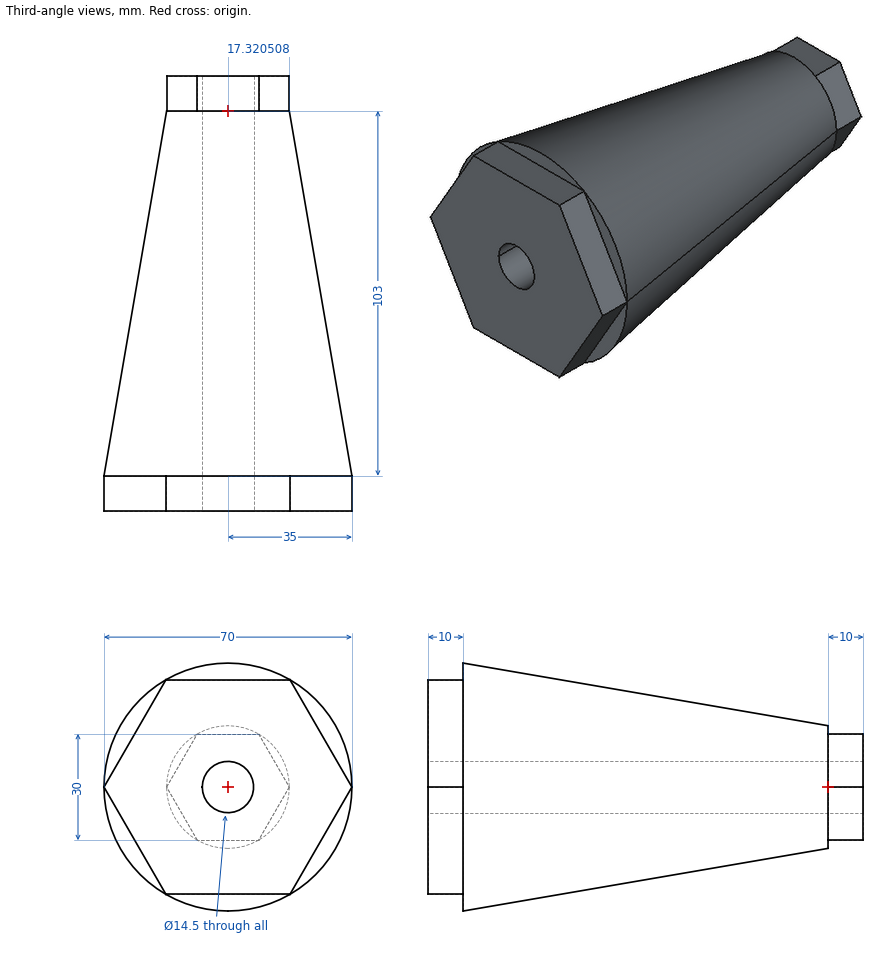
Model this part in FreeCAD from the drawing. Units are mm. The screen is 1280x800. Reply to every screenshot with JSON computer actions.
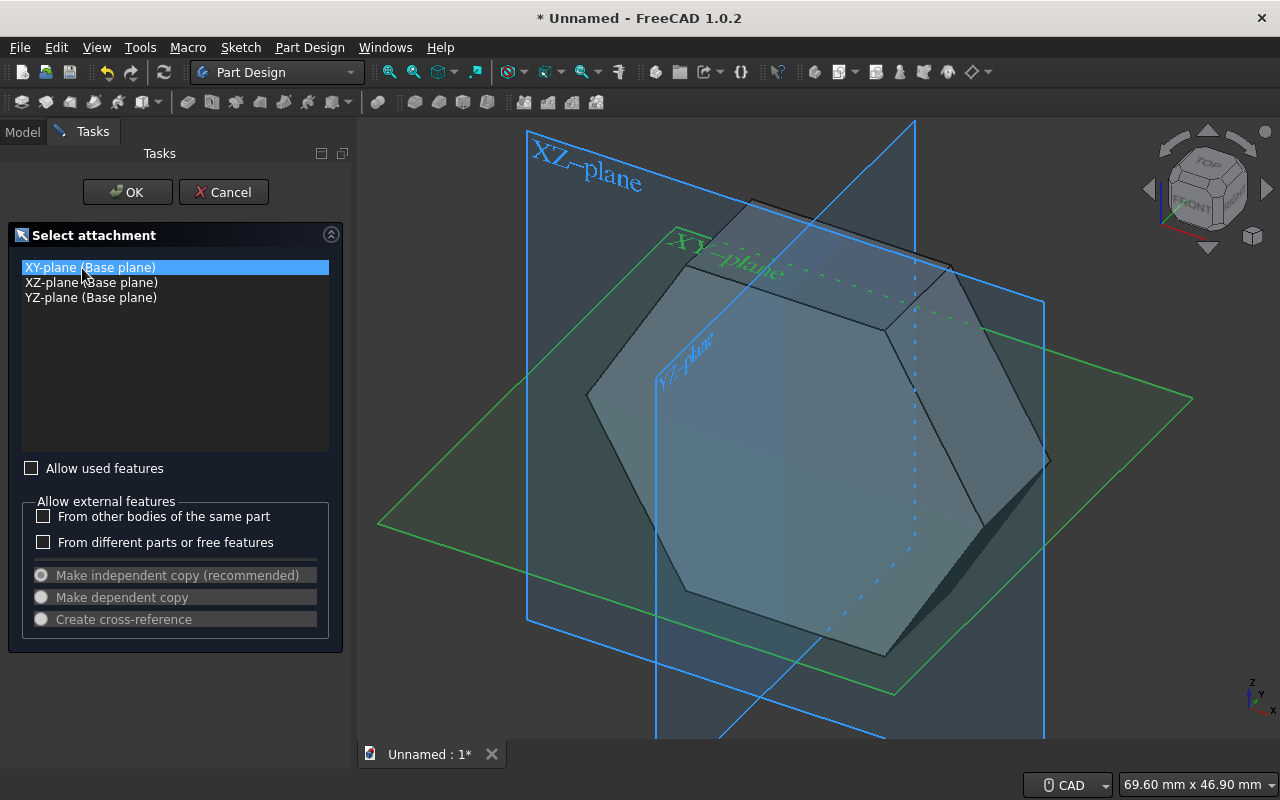
{"action": "left_click", "coordinate": [128, 192]}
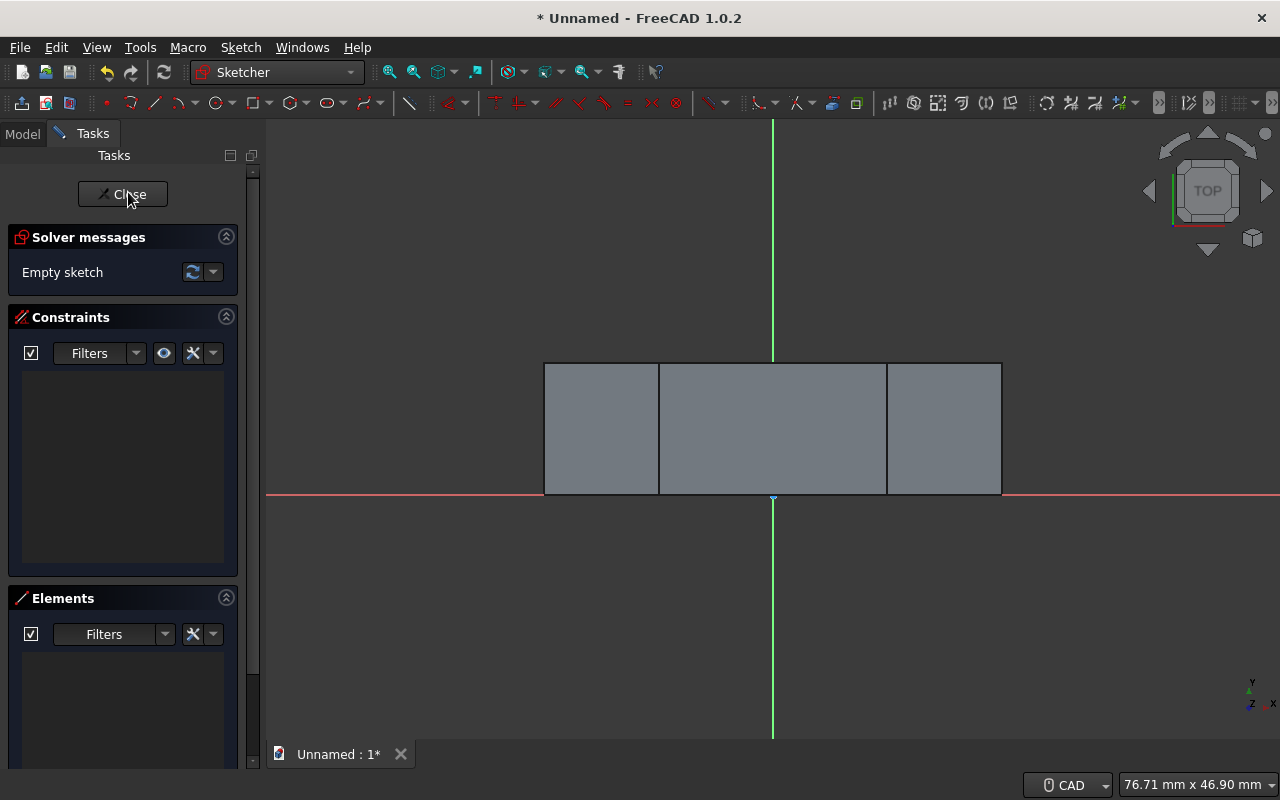
{"action": "left_click", "coordinate": [70, 104]}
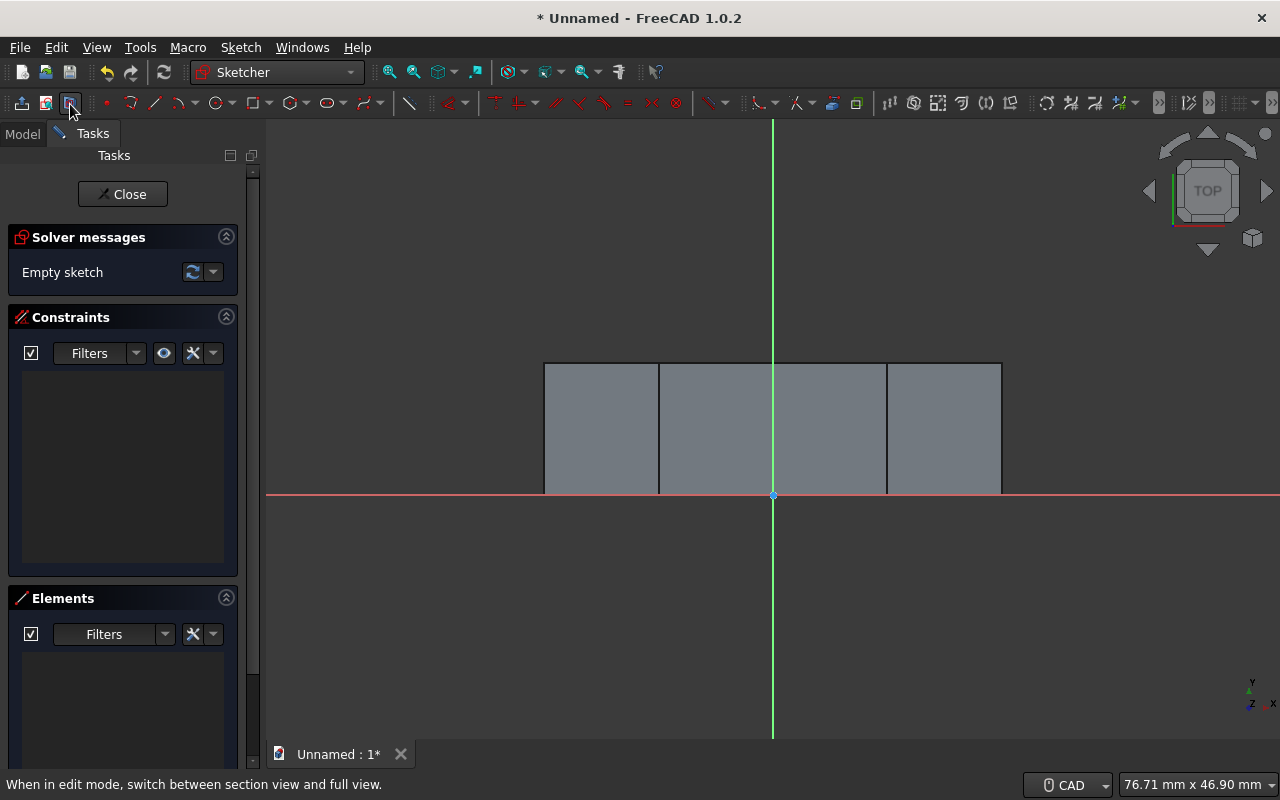
{"action": "scroll", "coordinate": [575, 147], "scroll_direction": "down", "scroll_amount": 6}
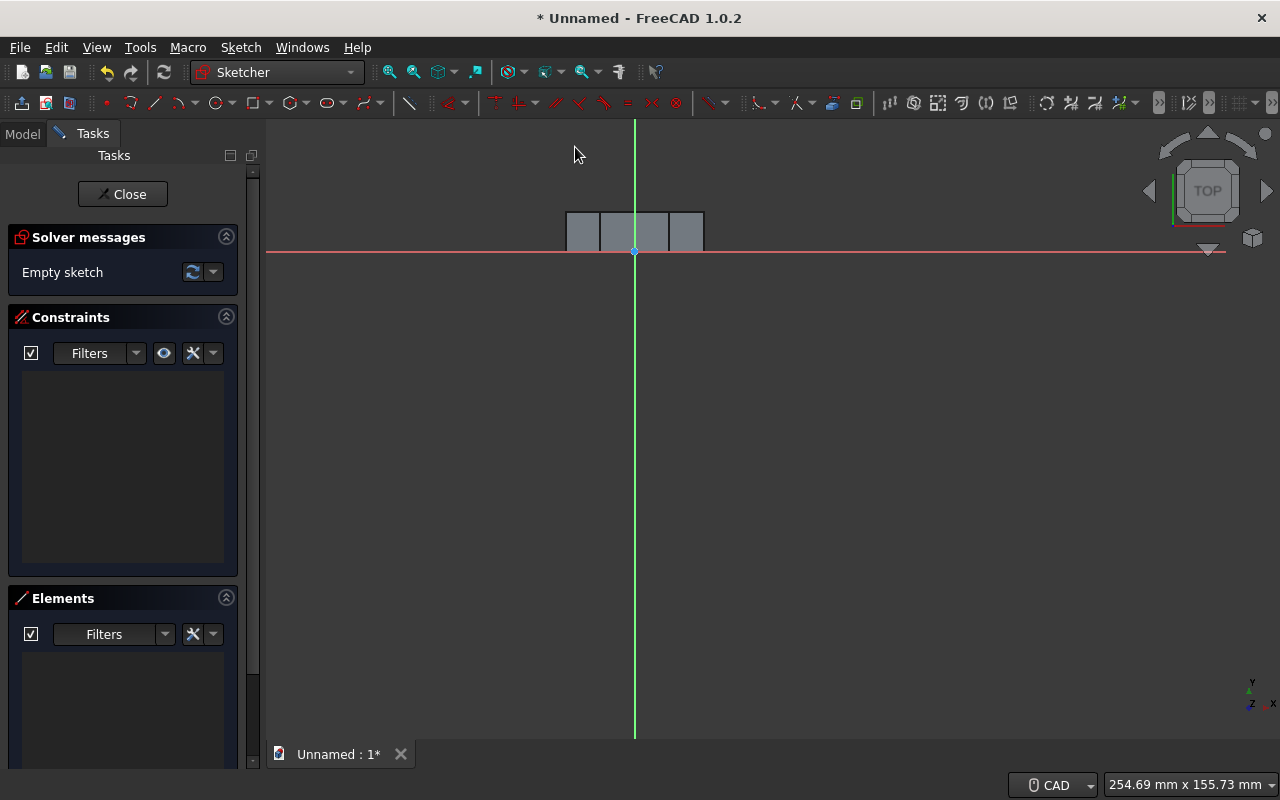
{"action": "left_click", "coordinate": [132, 104]}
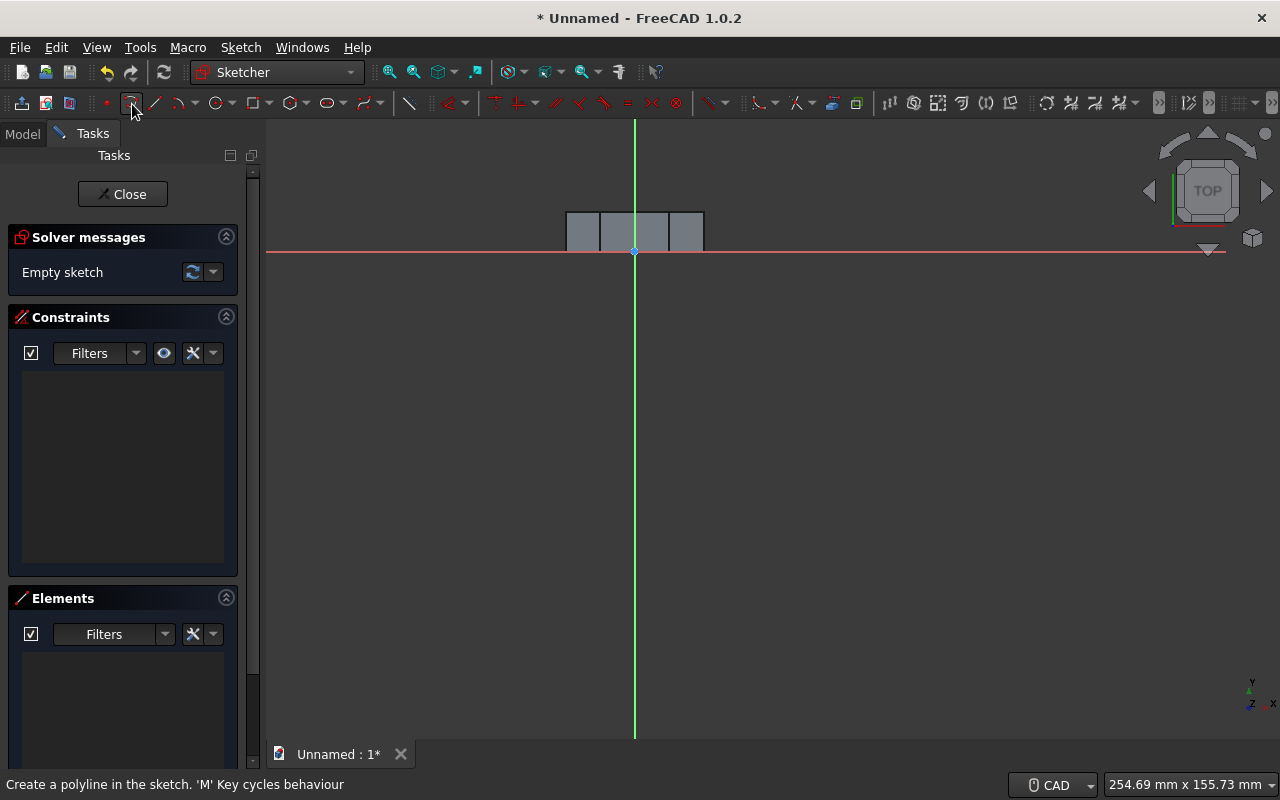
{"action": "left_click", "coordinate": [635, 252]}
{"action": "left_click", "coordinate": [644, 662]}
{"action": "left_click", "coordinate": [774, 662]}
{"action": "left_click", "coordinate": [704, 261]}
{"action": "left_click", "coordinate": [635, 252]}
{"action": "key", "text": "Escape"}
{"action": "key", "text": "Escape"}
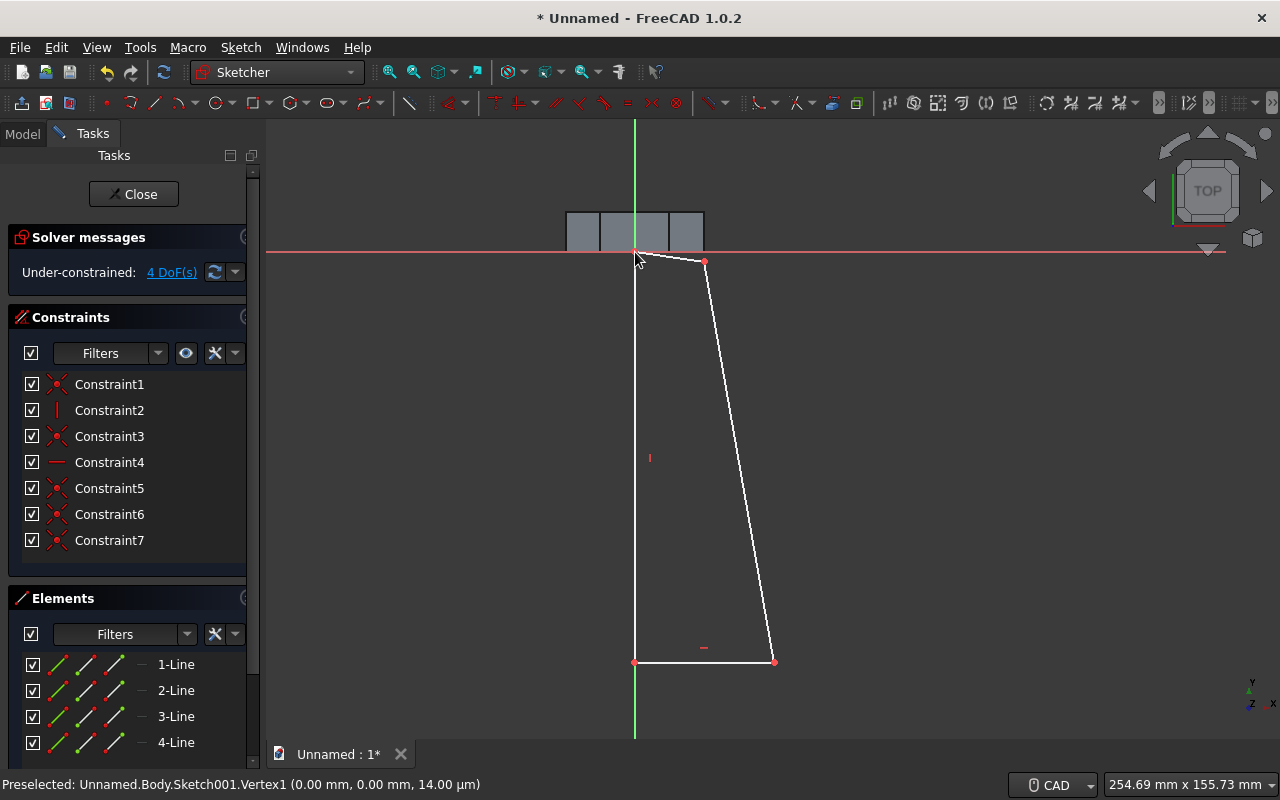
{"action": "left_click", "coordinate": [656, 255]}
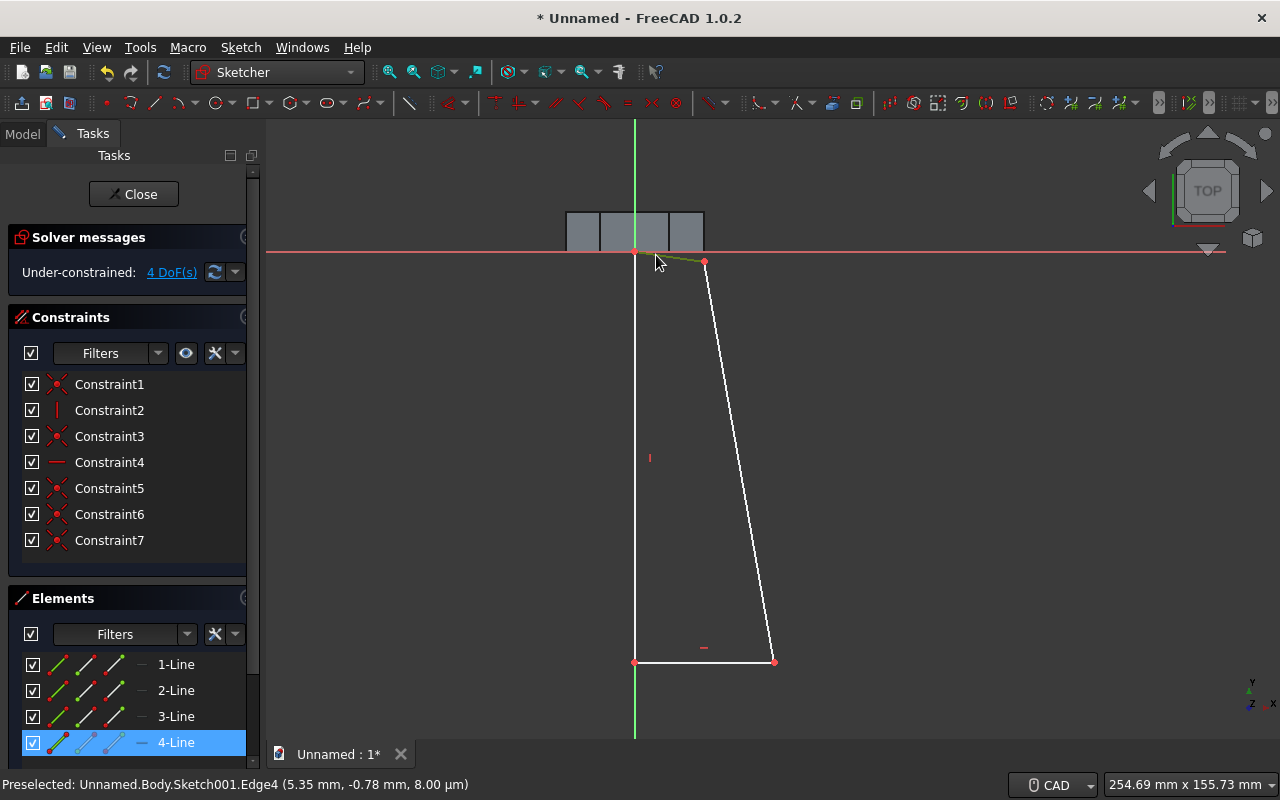
{"action": "left_click", "coordinate": [538, 104]}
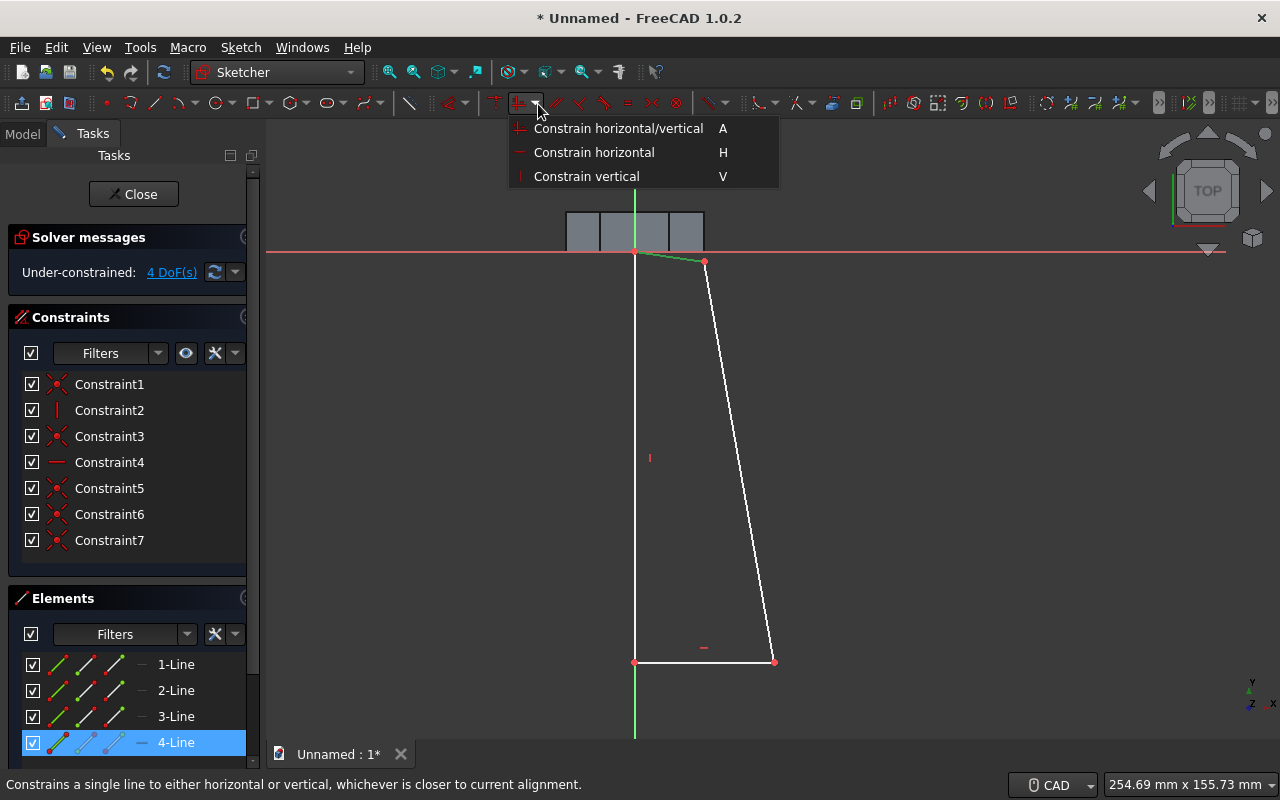
{"action": "left_click", "coordinate": [644, 152]}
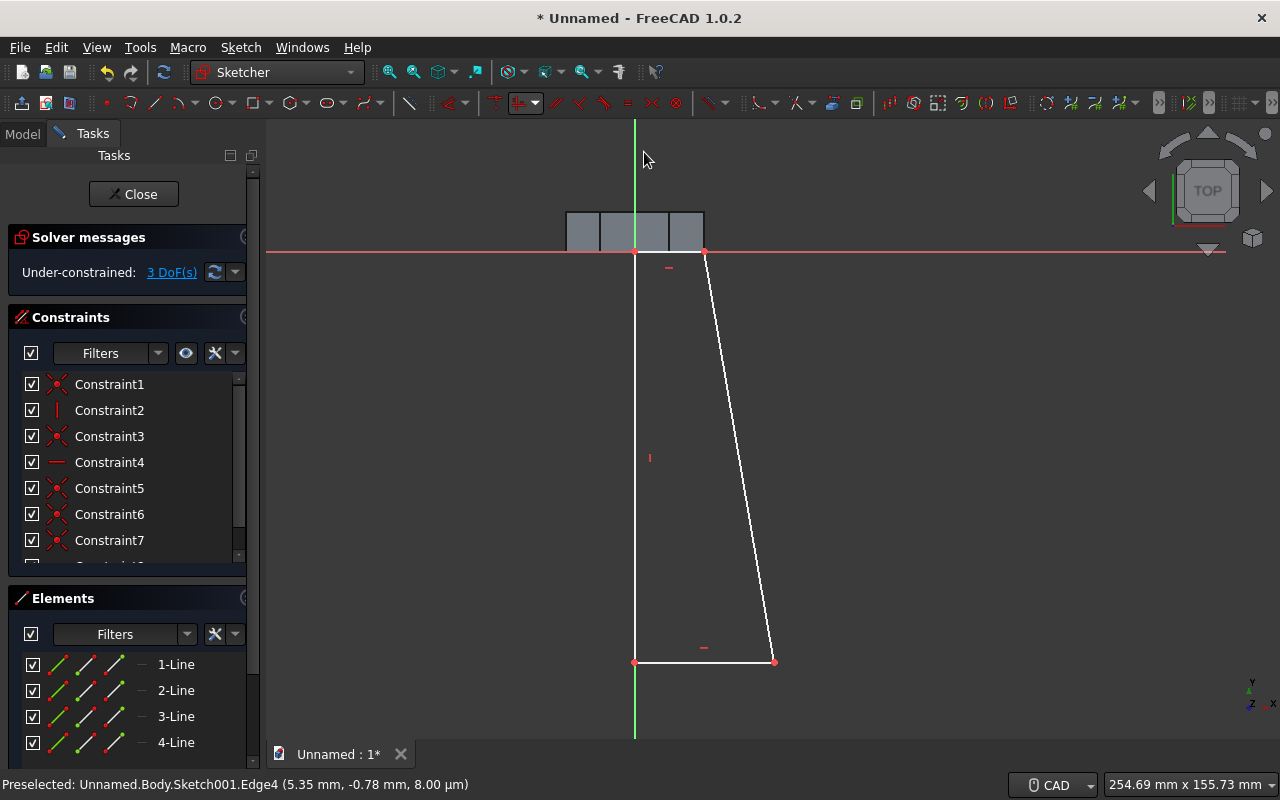
{"action": "left_click", "coordinate": [448, 104]}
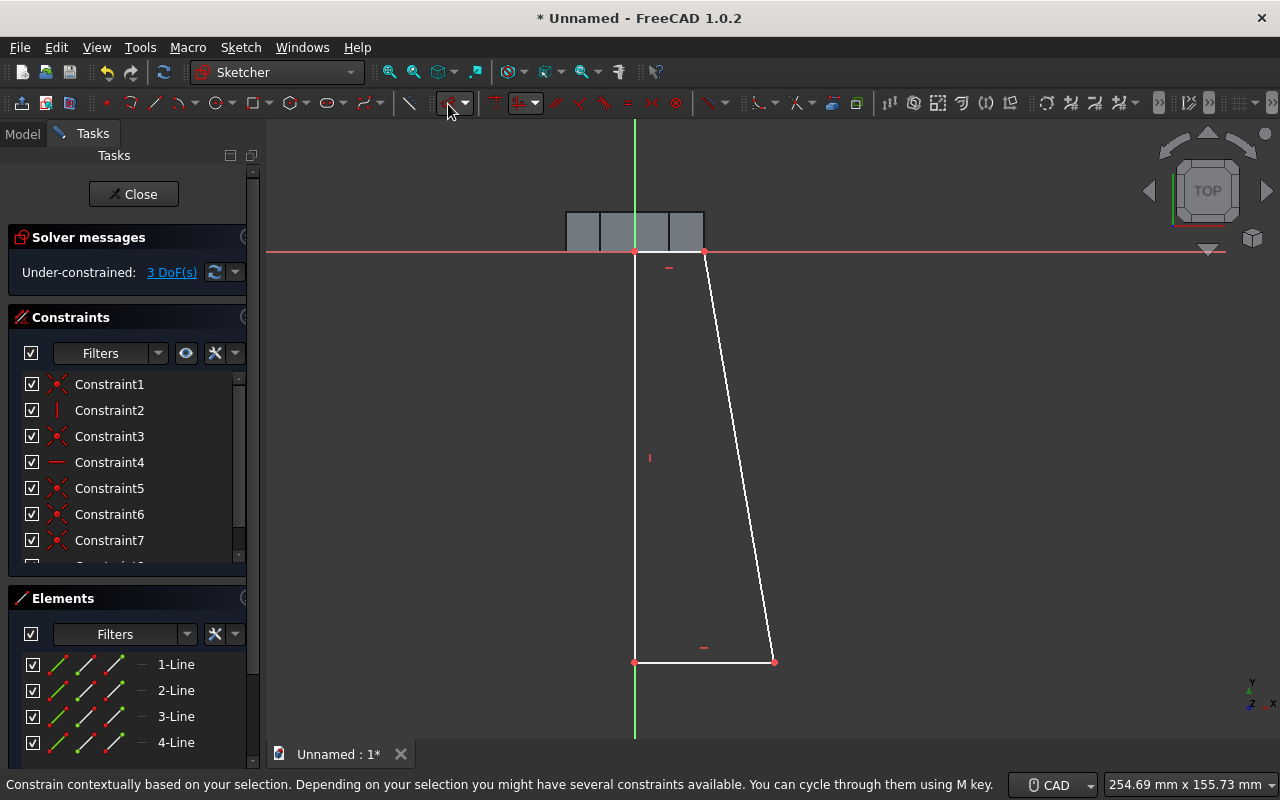
{"action": "left_click", "coordinate": [677, 663]}
{"action": "left_click", "coordinate": [704, 697]}